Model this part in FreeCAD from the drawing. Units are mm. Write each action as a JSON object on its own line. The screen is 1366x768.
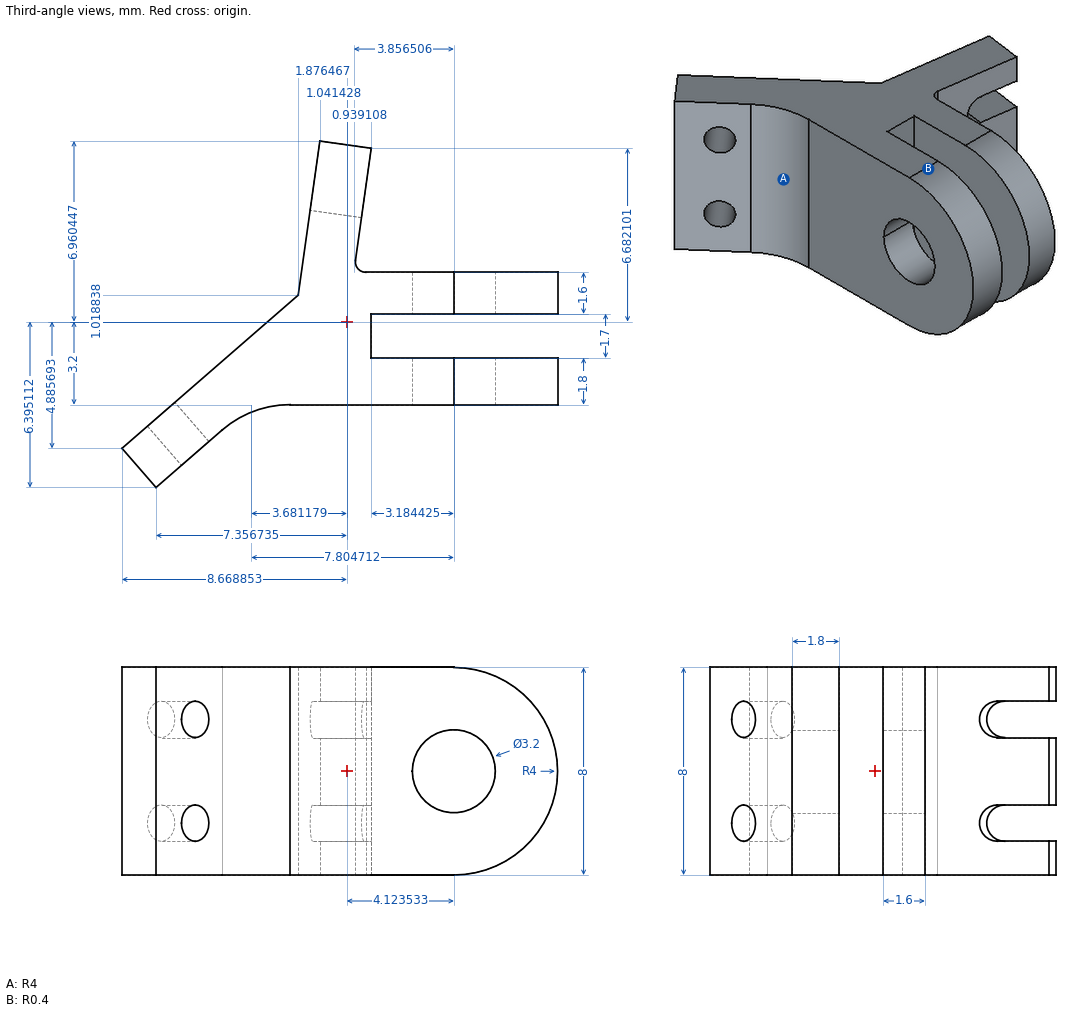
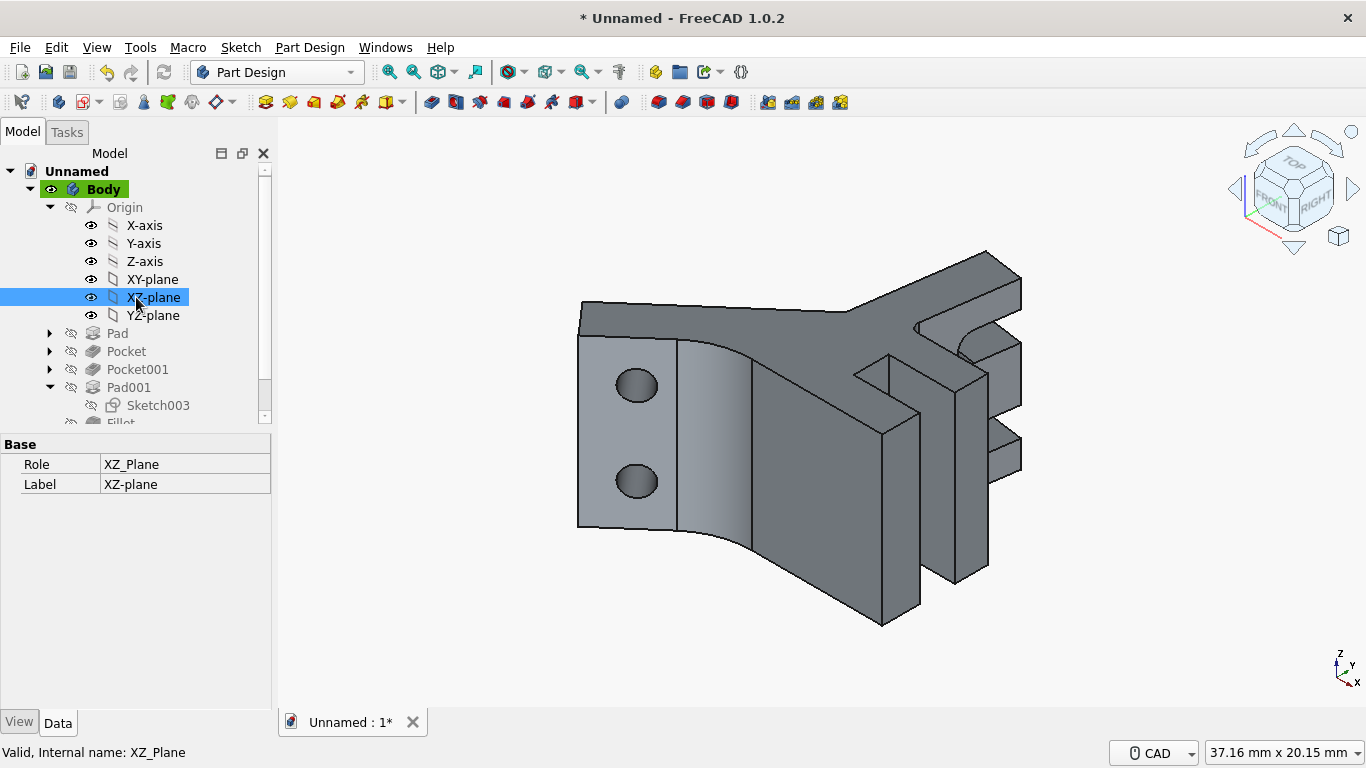
{"action": "left_click", "coordinate": [216, 102]}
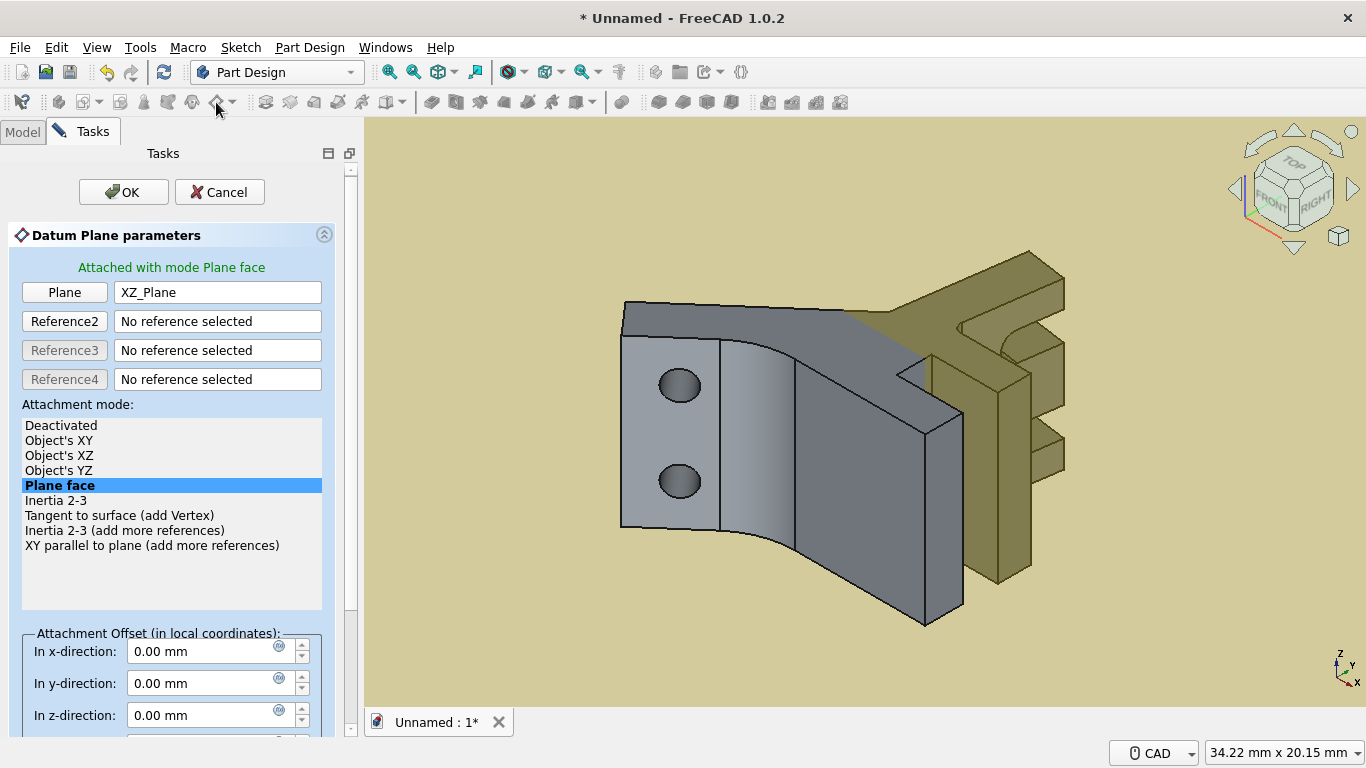
{"action": "triple_click", "coordinate": [210, 715]}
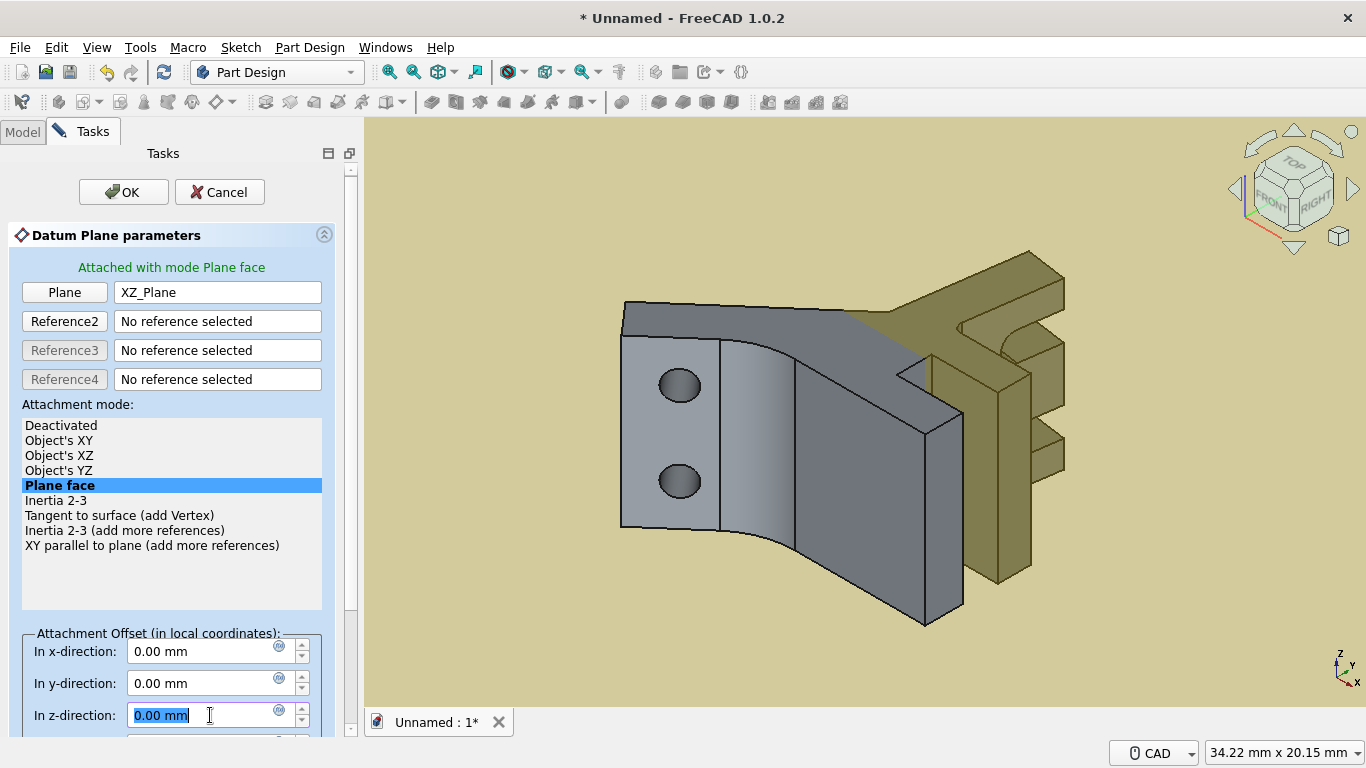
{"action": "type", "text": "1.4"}
{"action": "key", "text": "Tab"}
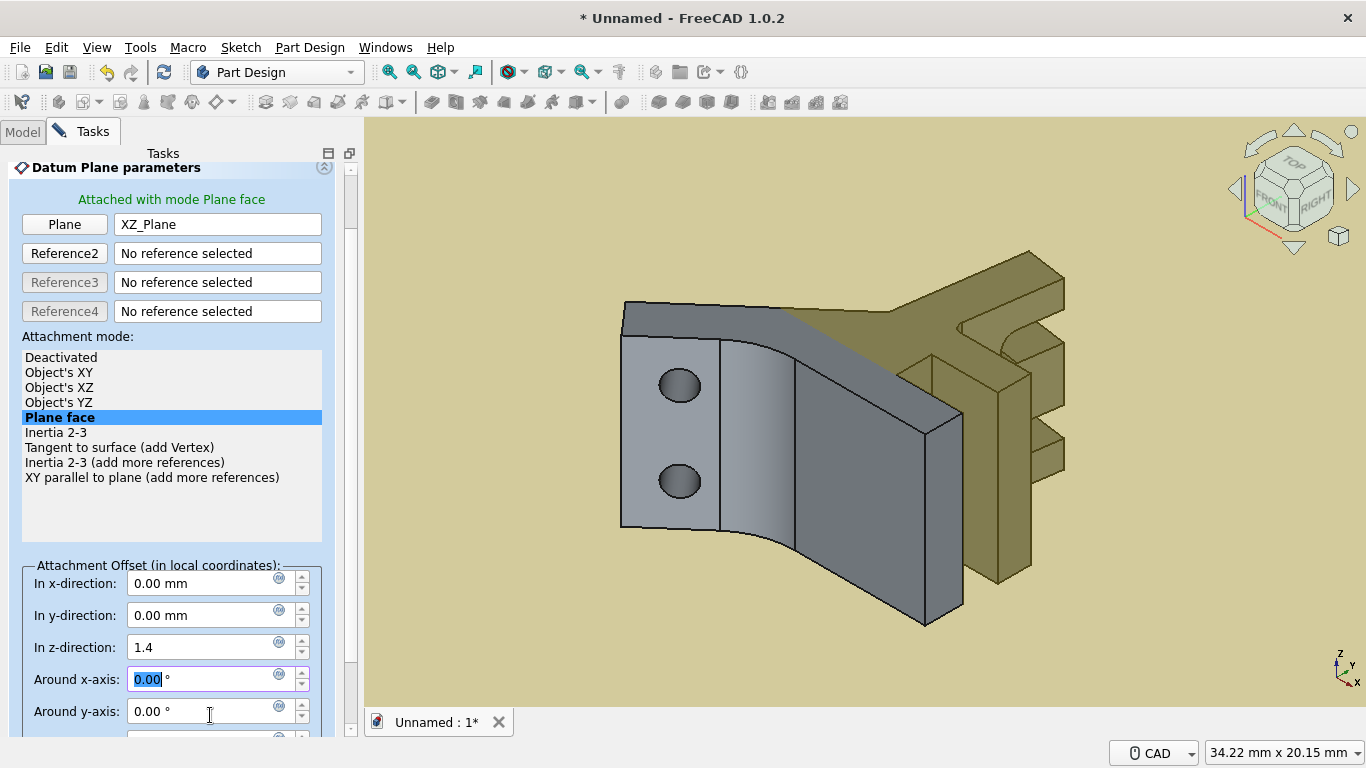
{"action": "scroll", "coordinate": [351, 450], "scroll_direction": "up", "scroll_amount": 2}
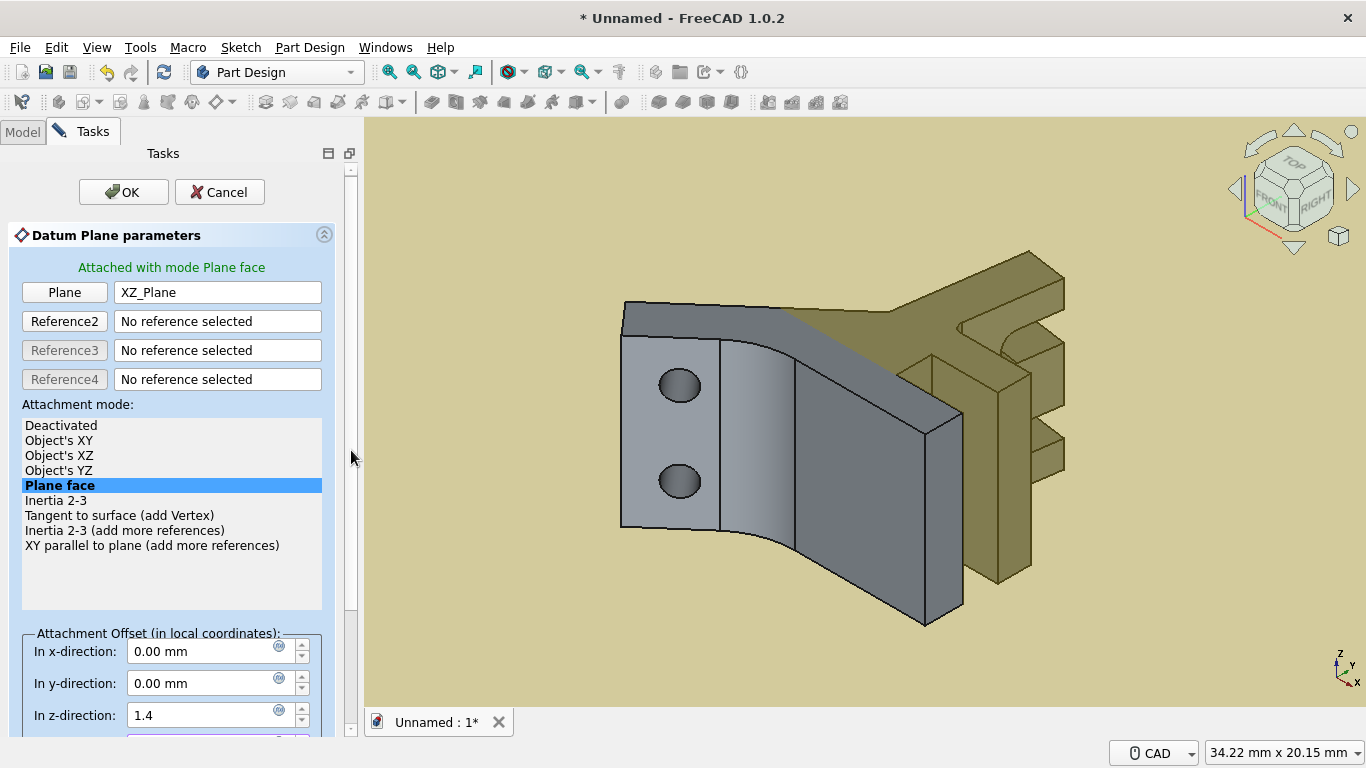
{"action": "left_click", "coordinate": [124, 192]}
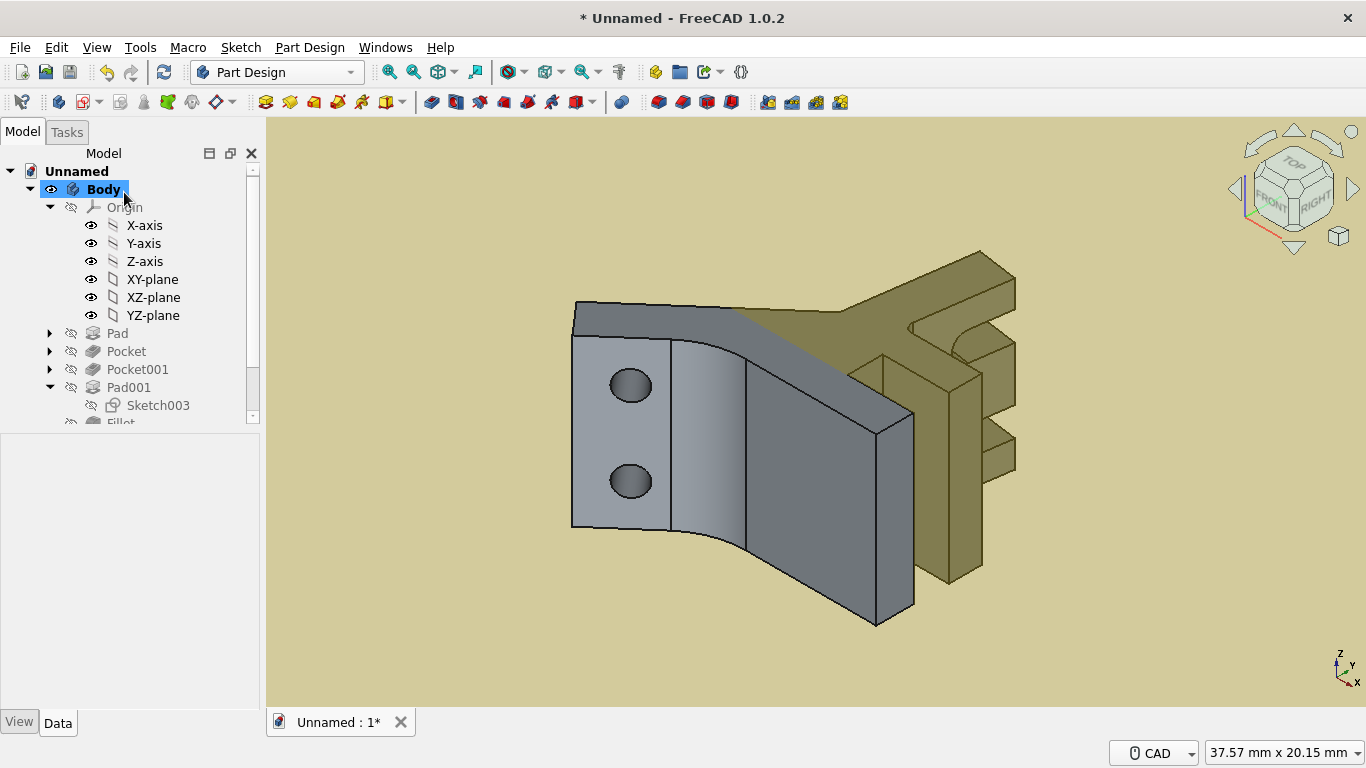
{"action": "scroll", "coordinate": [100, 293], "scroll_direction": "down", "scroll_amount": 3}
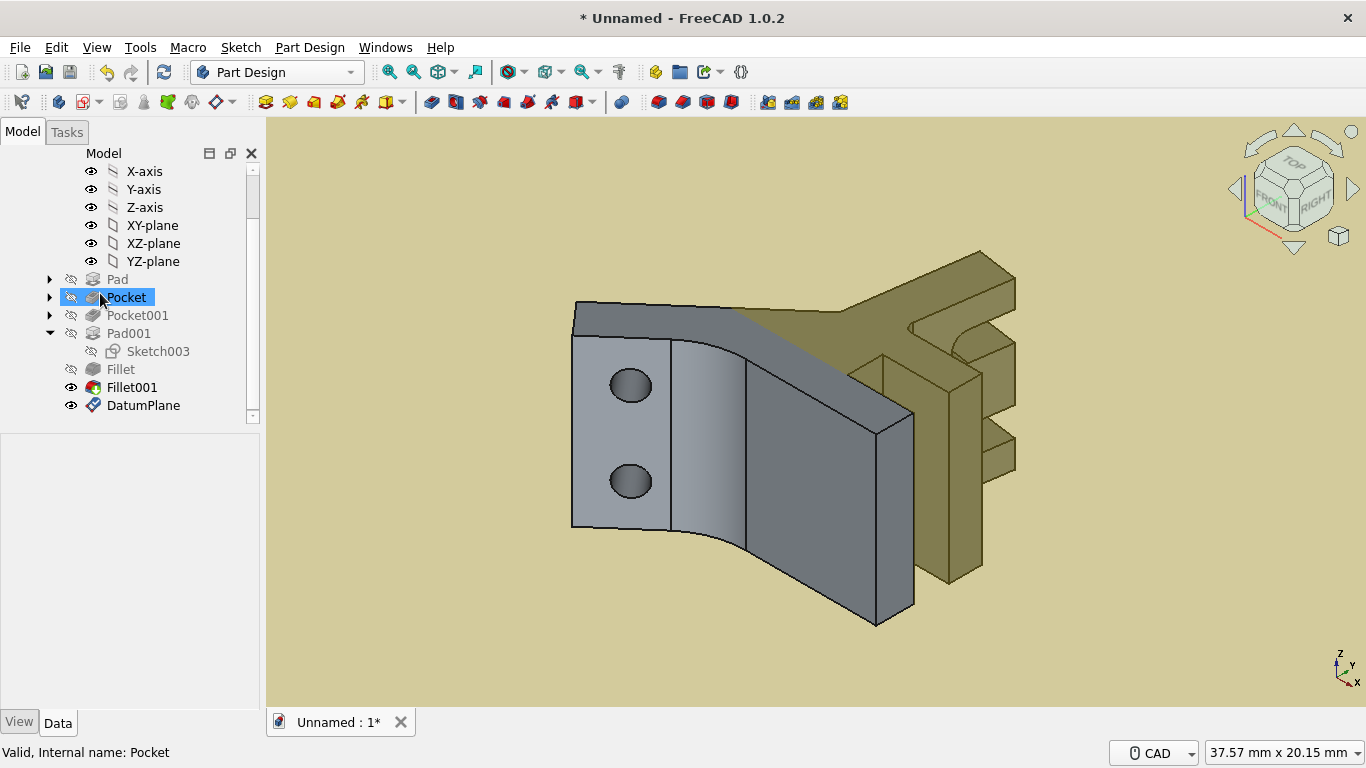
{"action": "left_click", "coordinate": [116, 405]}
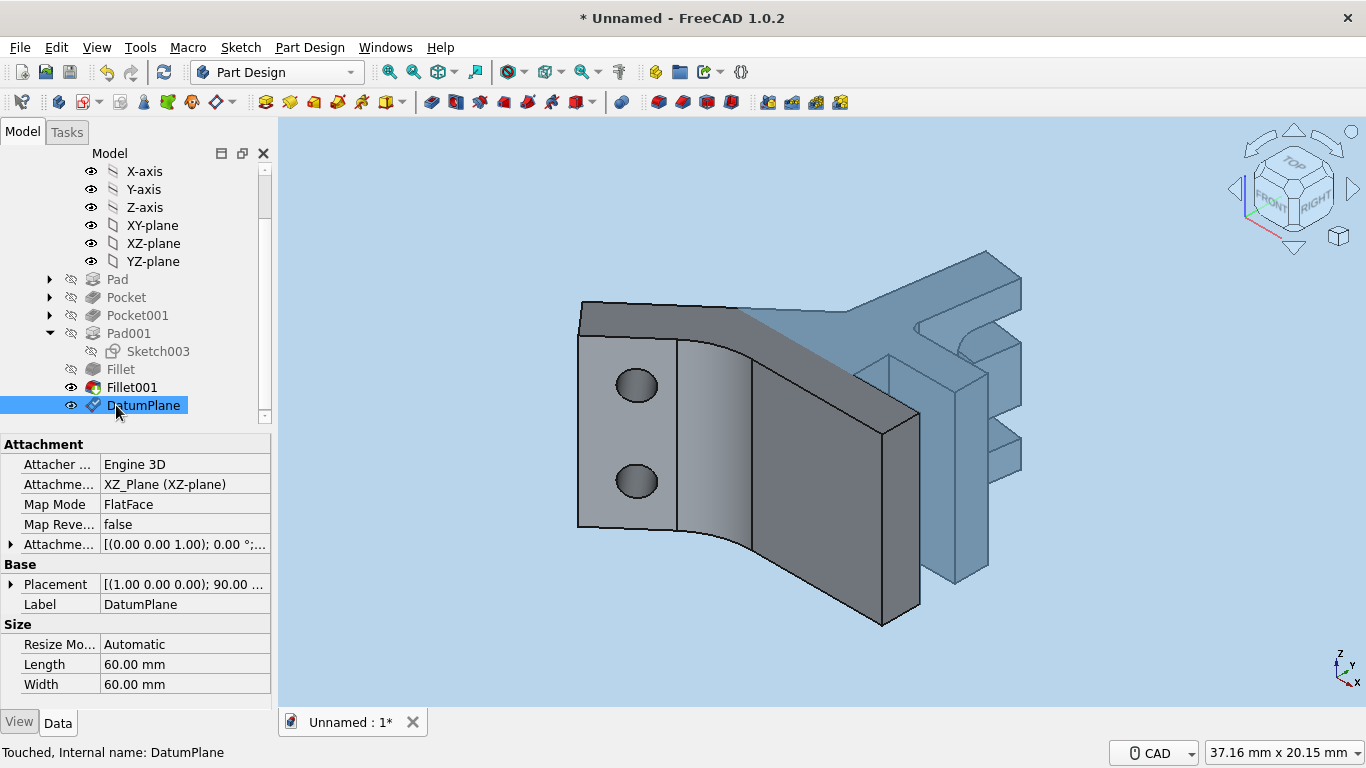
{"action": "left_click", "coordinate": [84, 102]}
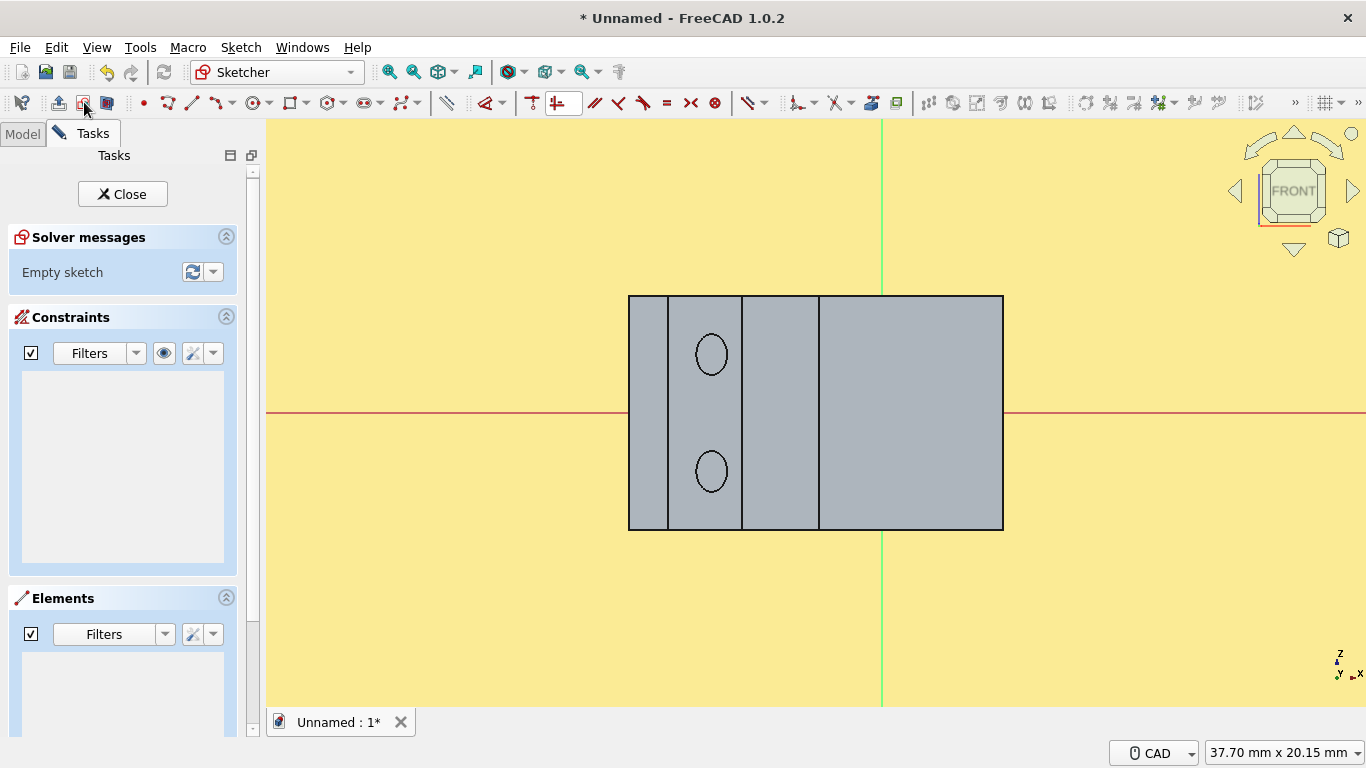
{"action": "left_click", "coordinate": [108, 104]}